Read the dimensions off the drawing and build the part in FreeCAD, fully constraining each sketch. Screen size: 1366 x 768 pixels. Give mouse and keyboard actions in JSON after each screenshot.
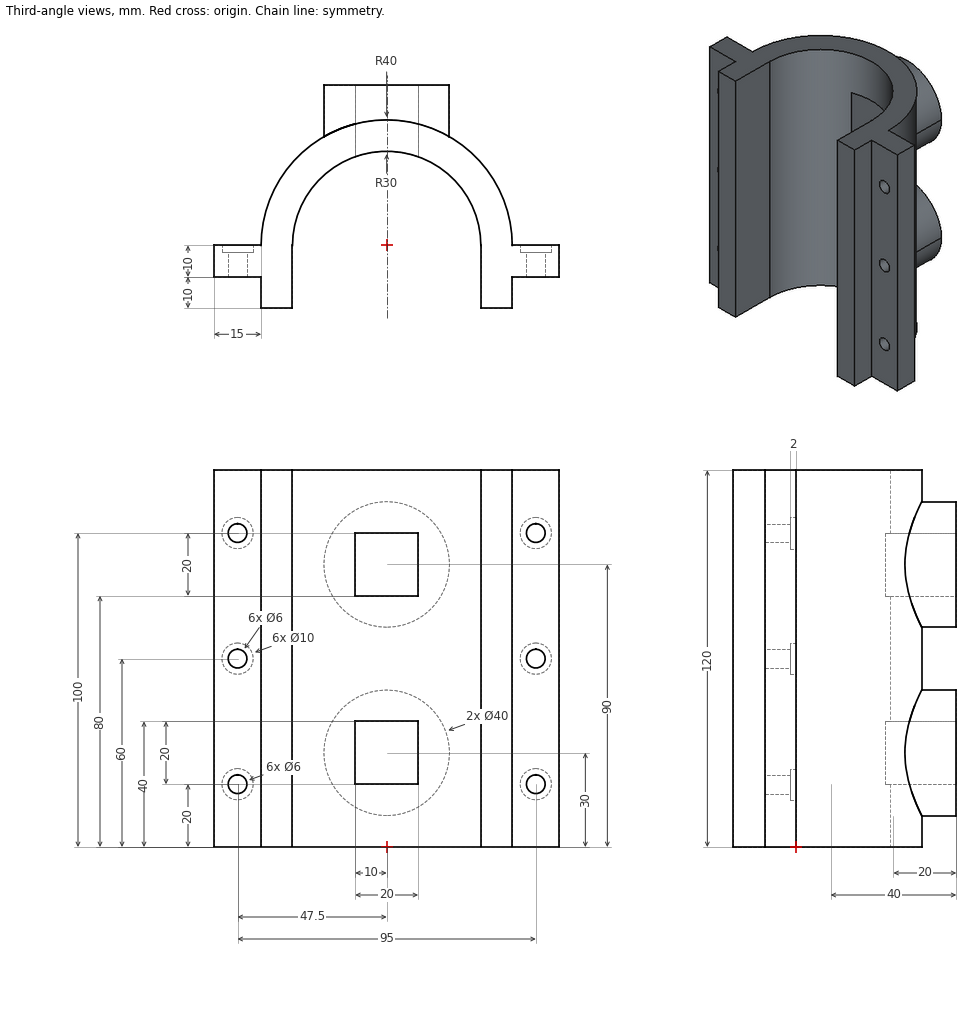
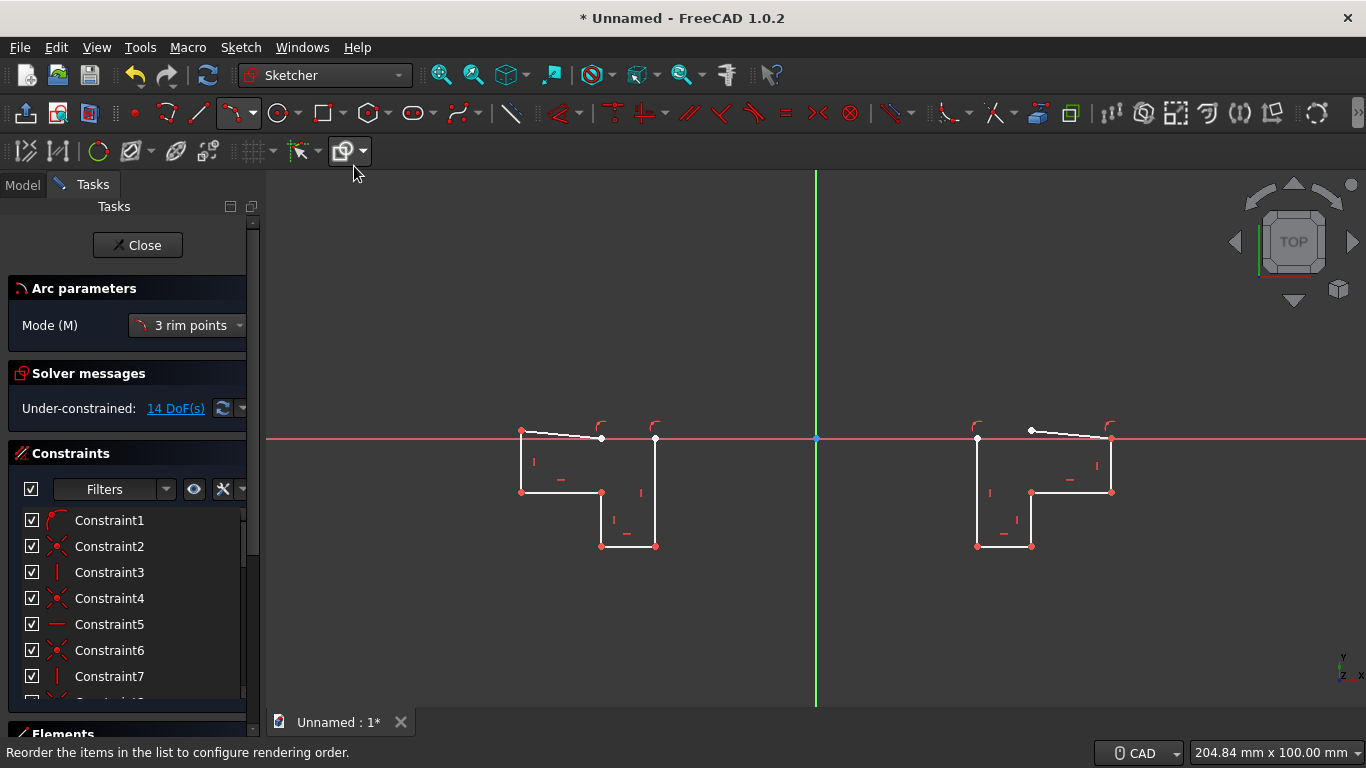
{"action": "left_click", "coordinate": [655, 438]}
{"action": "left_click", "coordinate": [977, 438]}
{"action": "left_click", "coordinate": [866, 285]}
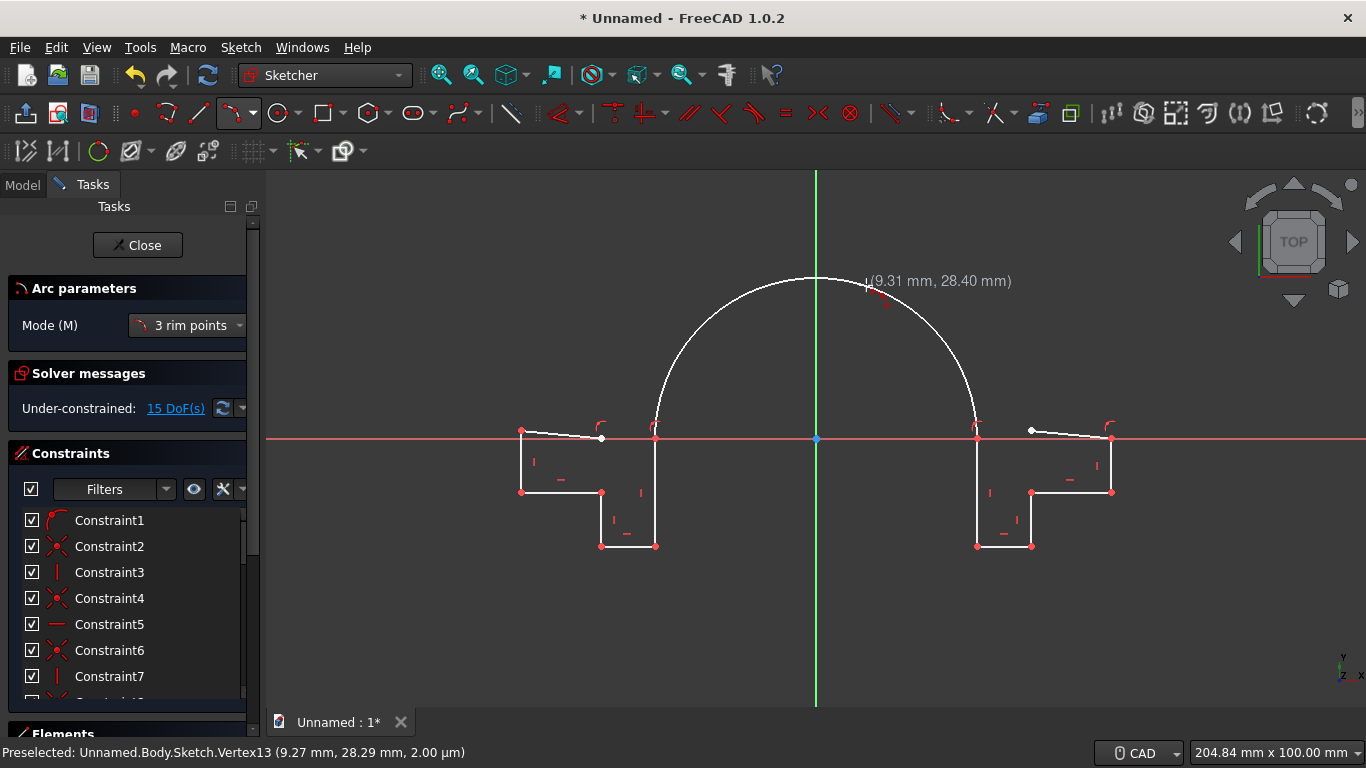
{"action": "left_click", "coordinate": [1031, 431]}
{"action": "left_click", "coordinate": [601, 438]}
{"action": "left_click", "coordinate": [882, 234]}
{"action": "key", "text": "Escape"}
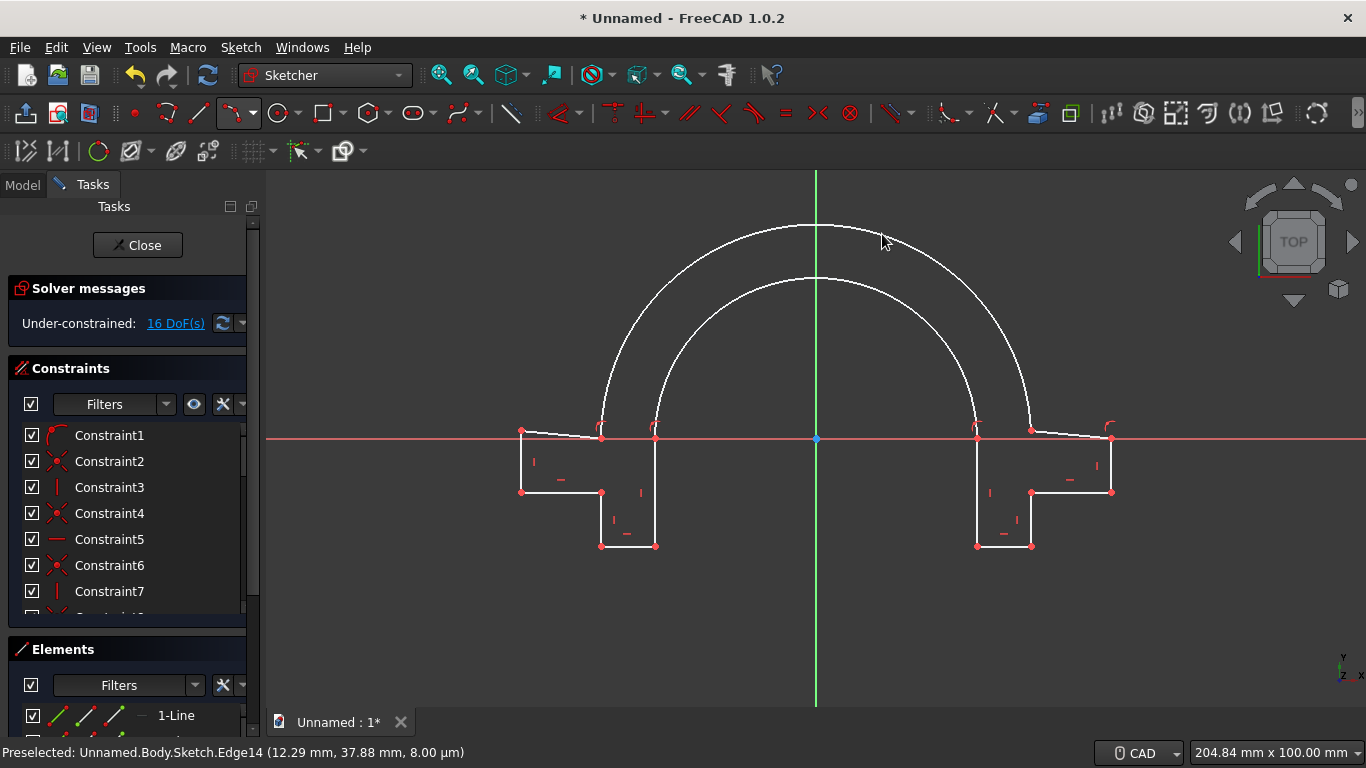
{"action": "left_click", "coordinate": [577, 436]}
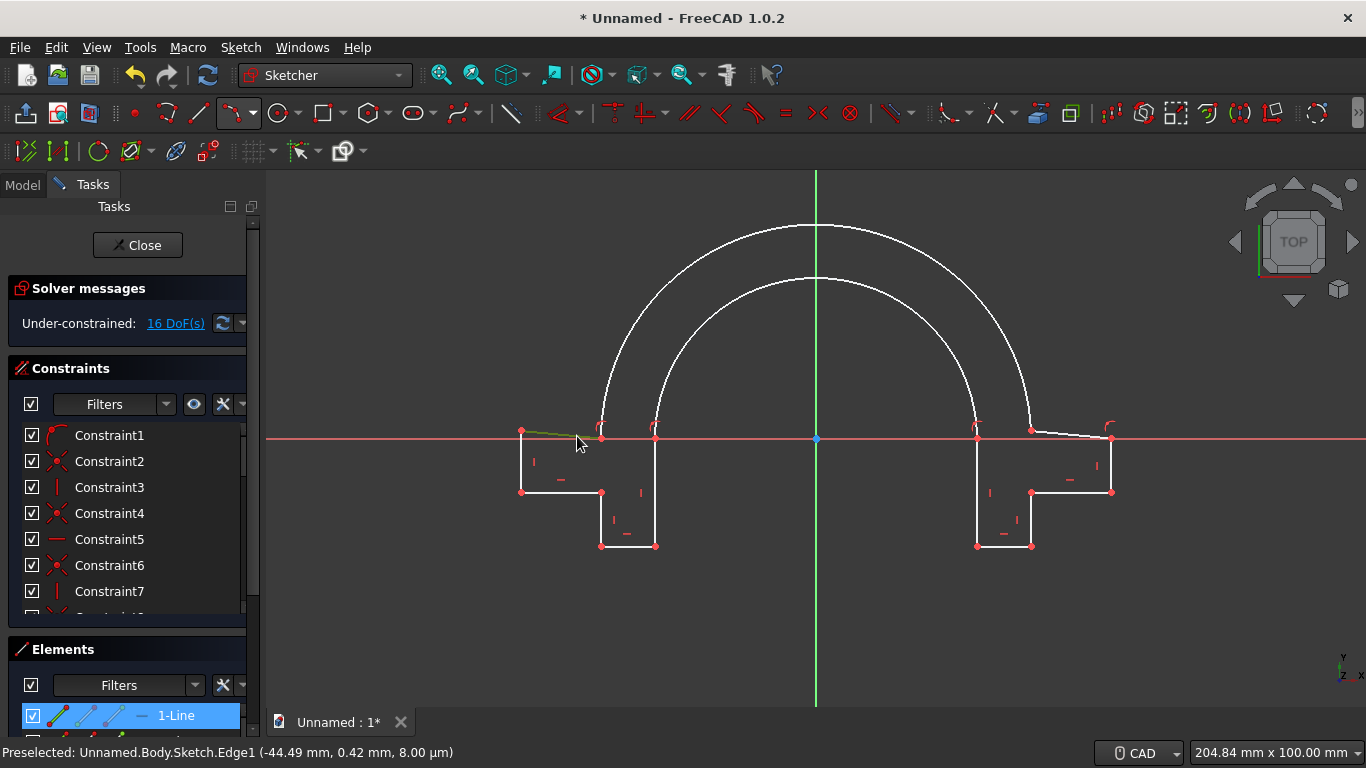
{"action": "left_click", "coordinate": [668, 114]}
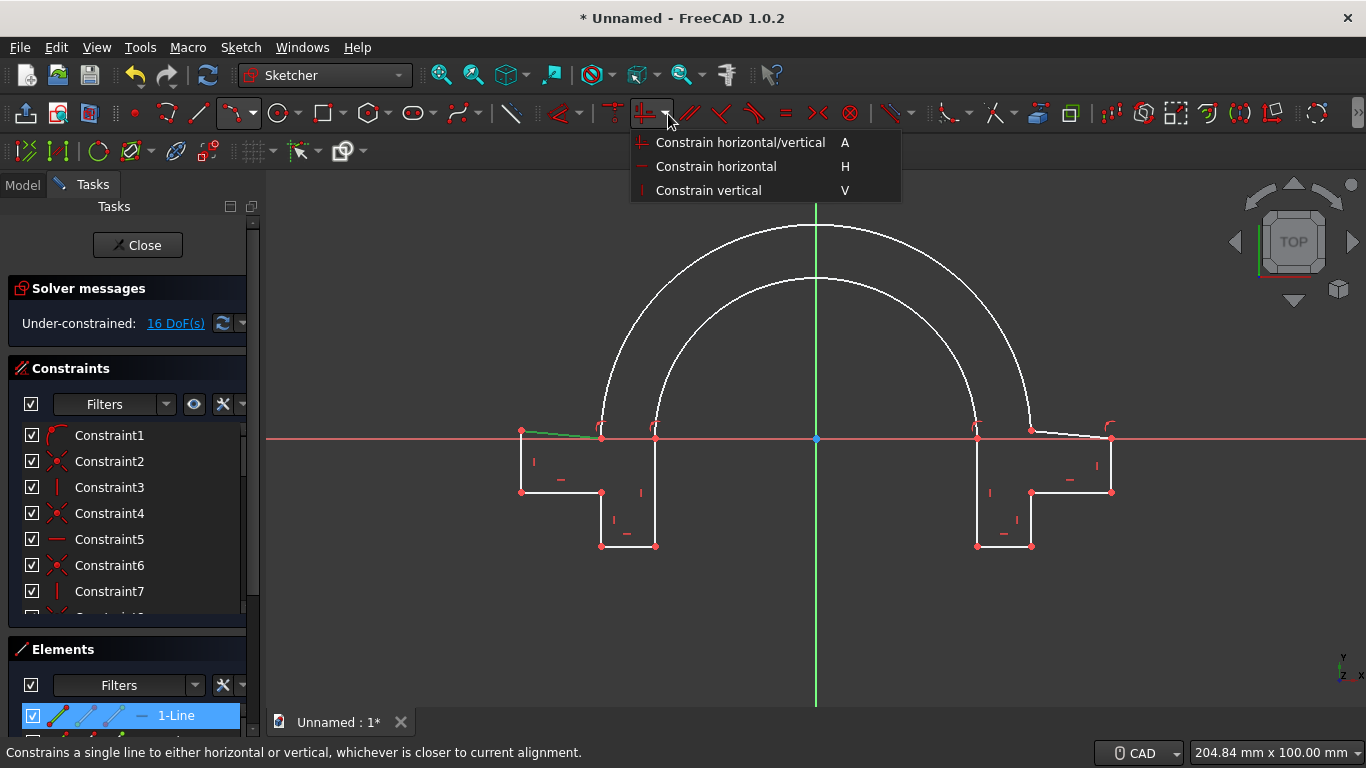
{"action": "left_click", "coordinate": [766, 166]}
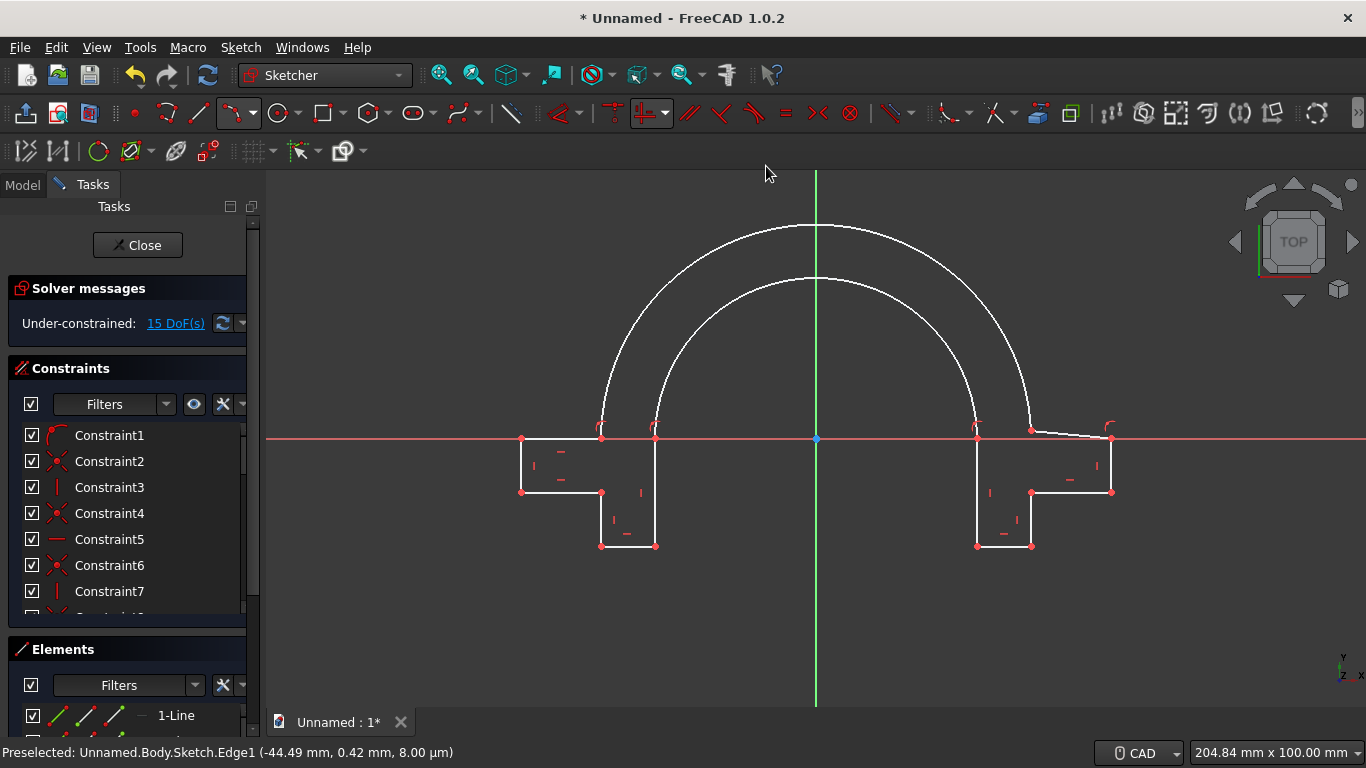
{"action": "left_click", "coordinate": [1087, 436]}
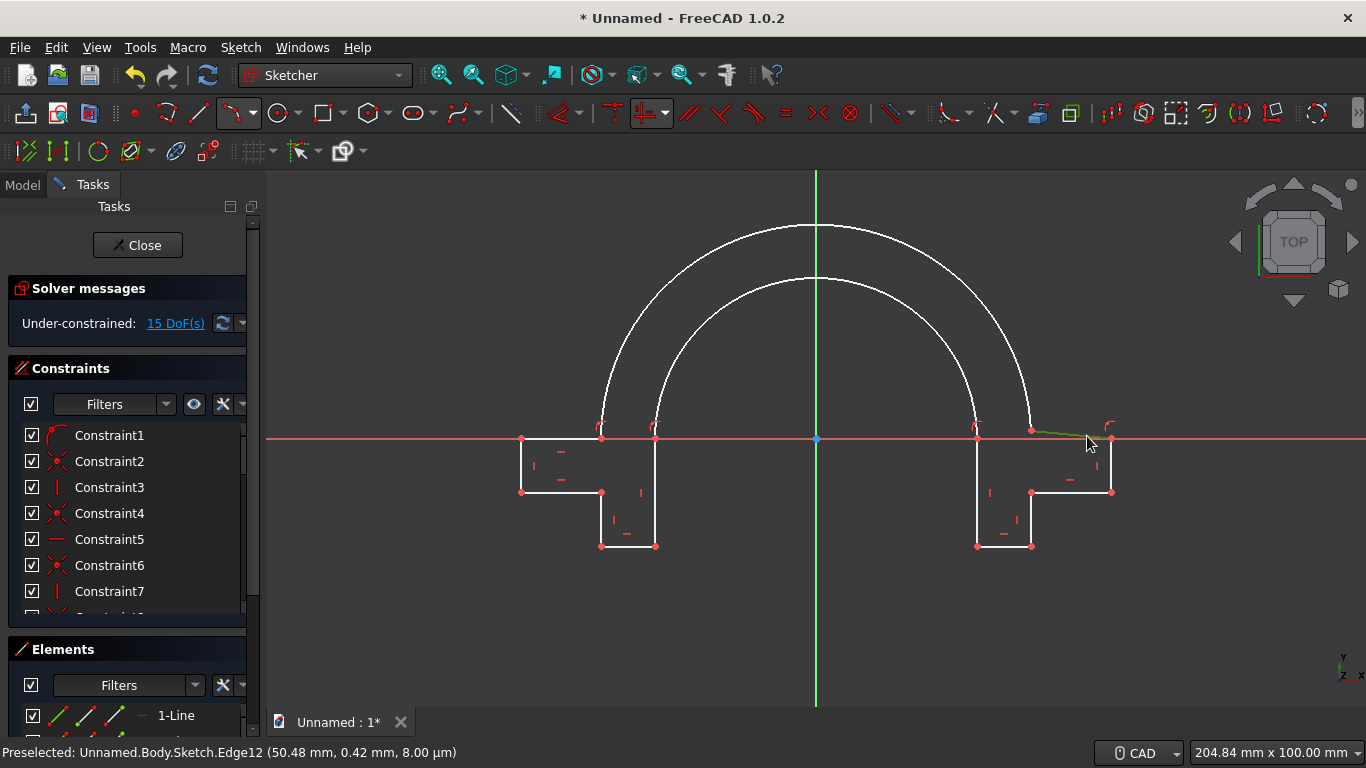
{"action": "key", "text": "h"}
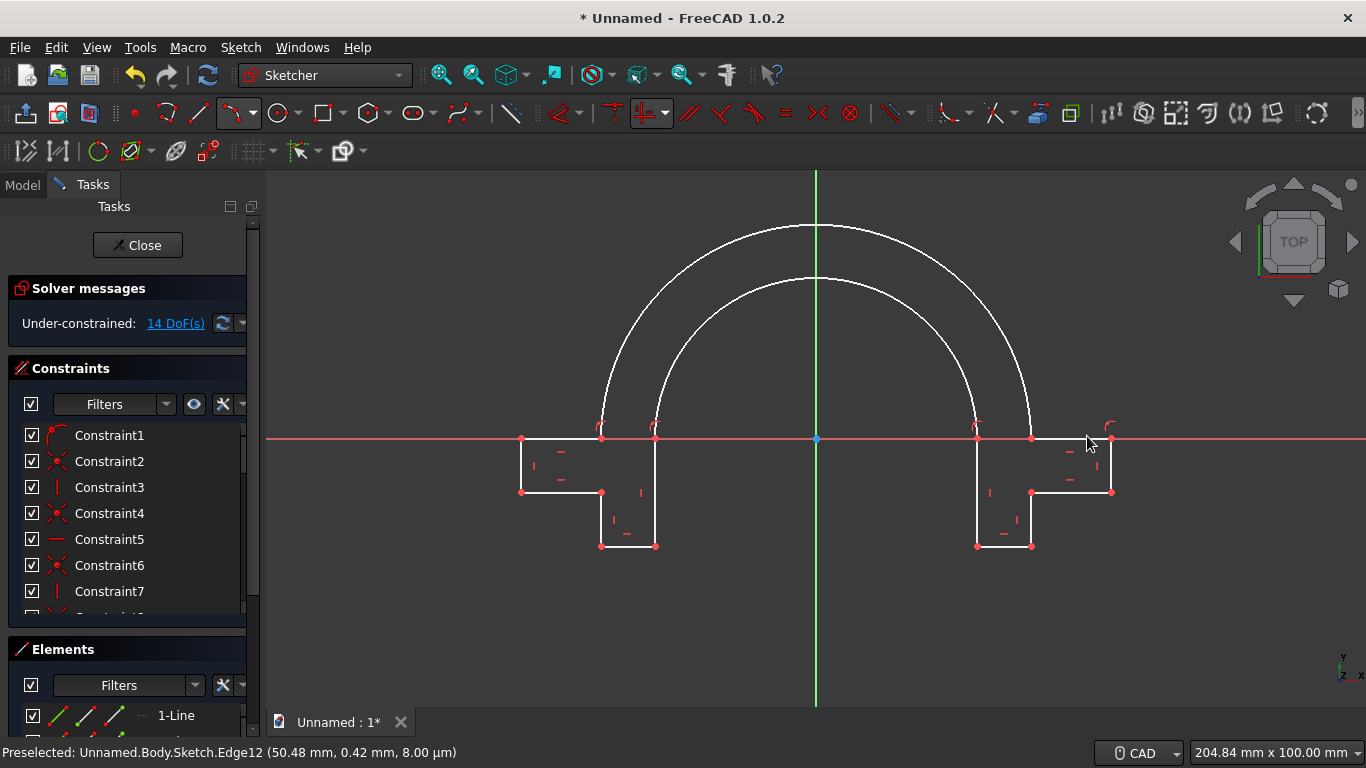
{"action": "left_click", "coordinate": [910, 309]}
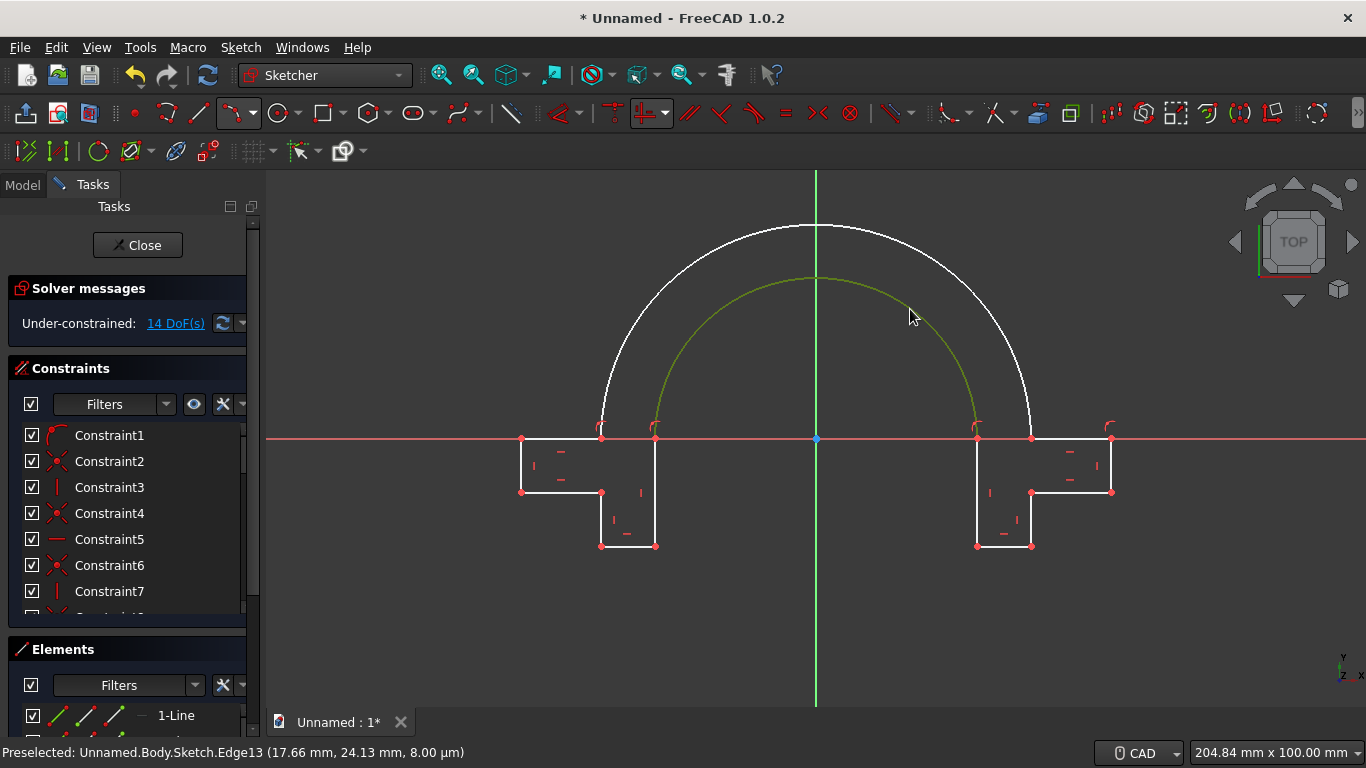
{"action": "left_click", "coordinate": [942, 266]}